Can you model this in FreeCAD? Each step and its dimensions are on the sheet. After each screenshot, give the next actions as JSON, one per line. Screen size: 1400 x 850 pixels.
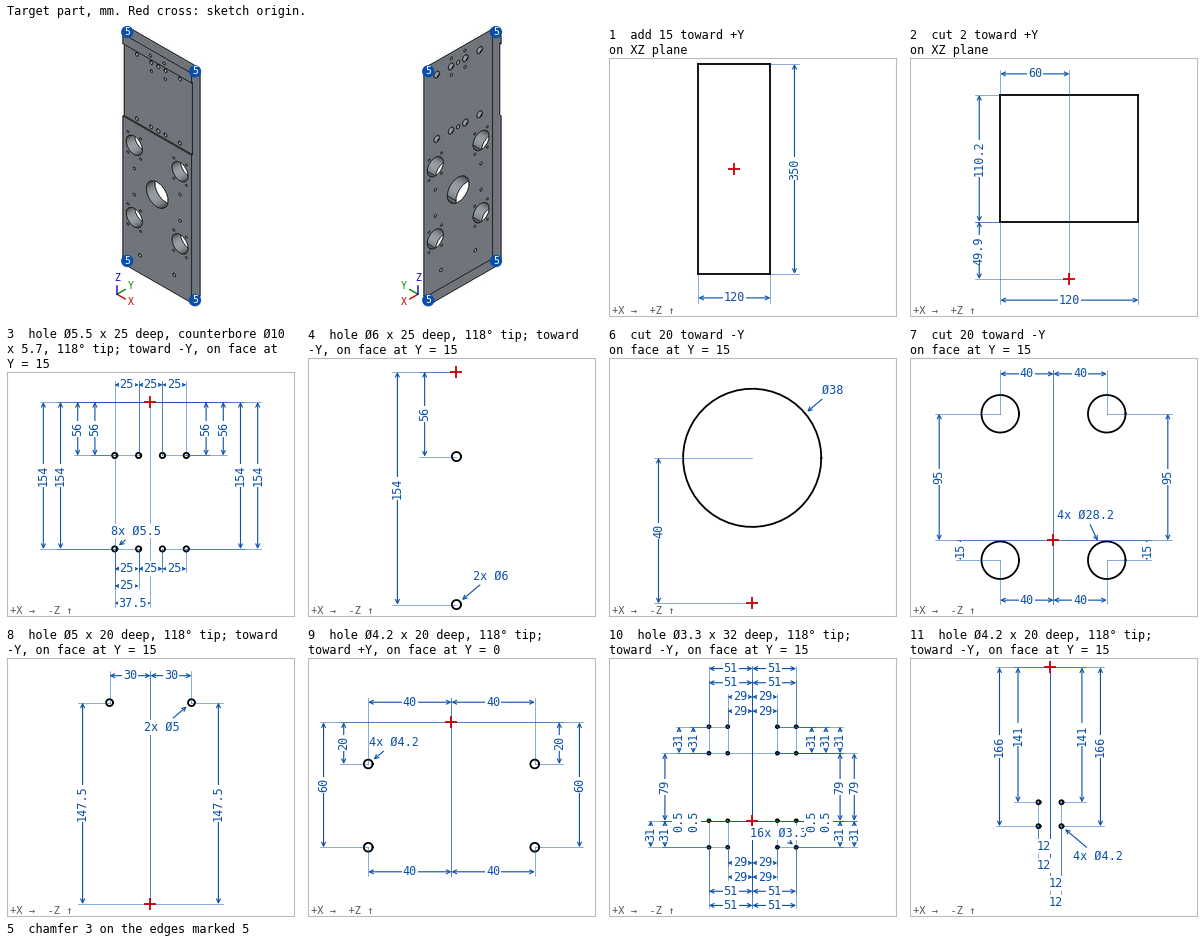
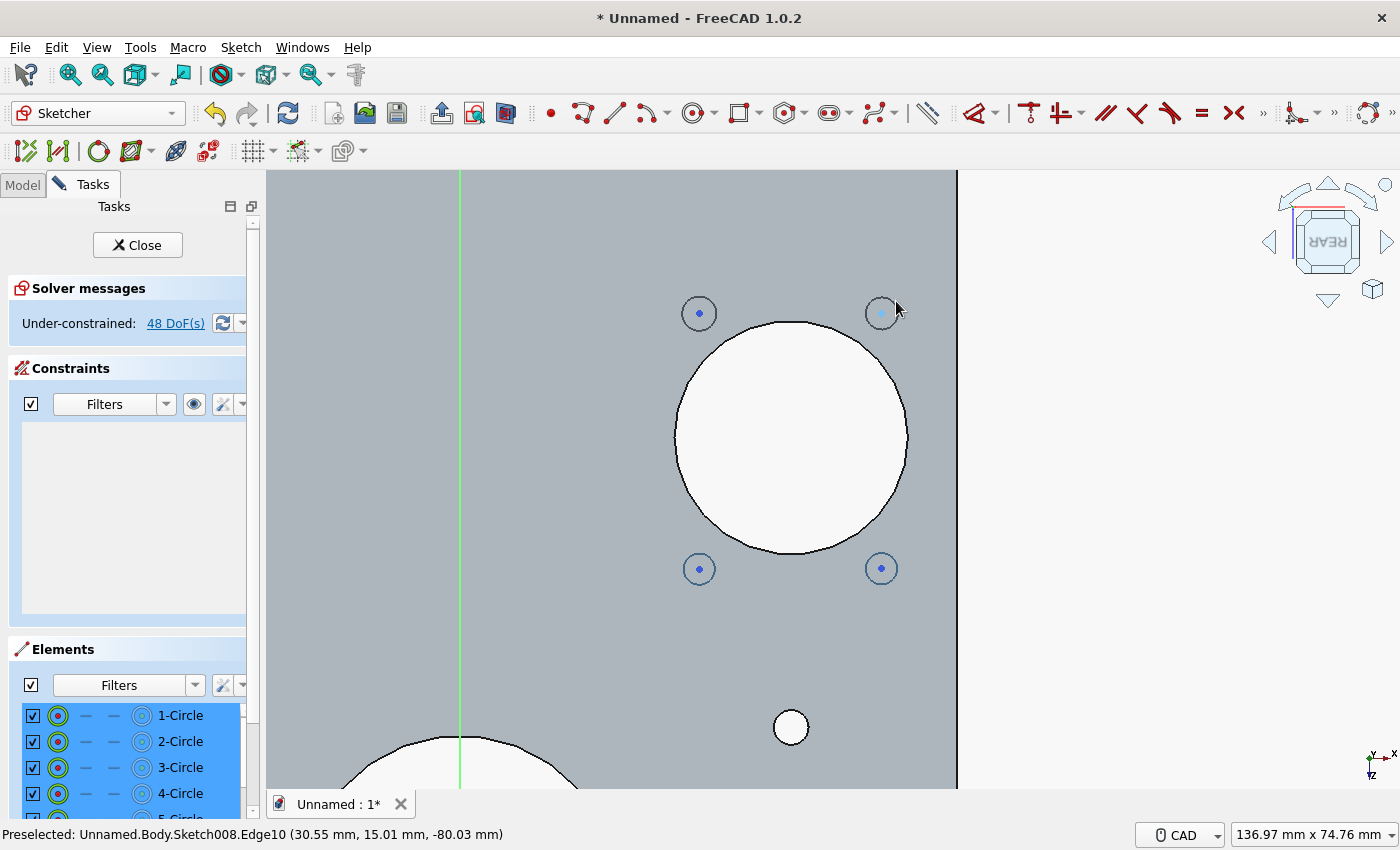
{"action": "left_click", "coordinate": [893, 302]}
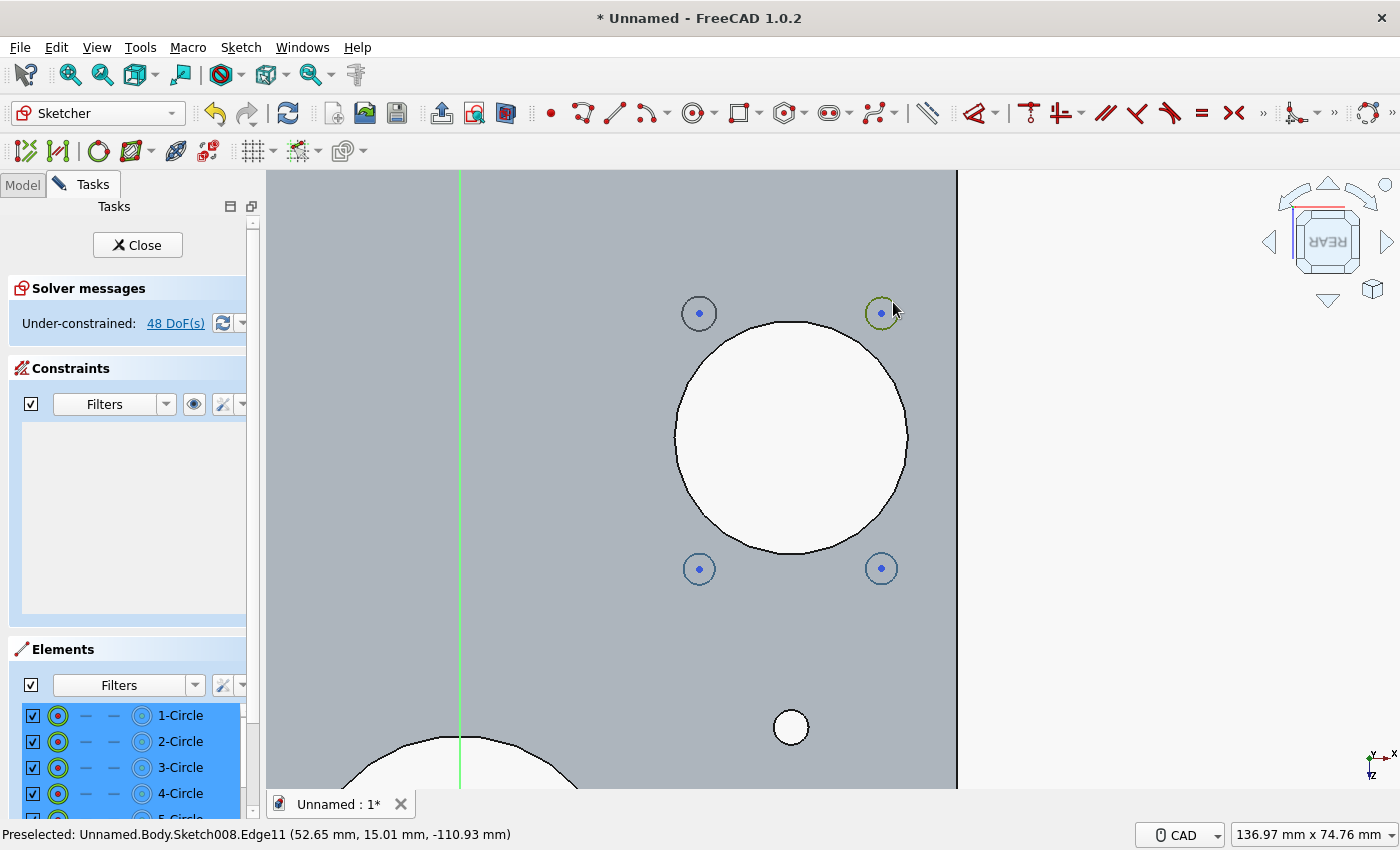
{"action": "left_click", "coordinate": [711, 302]}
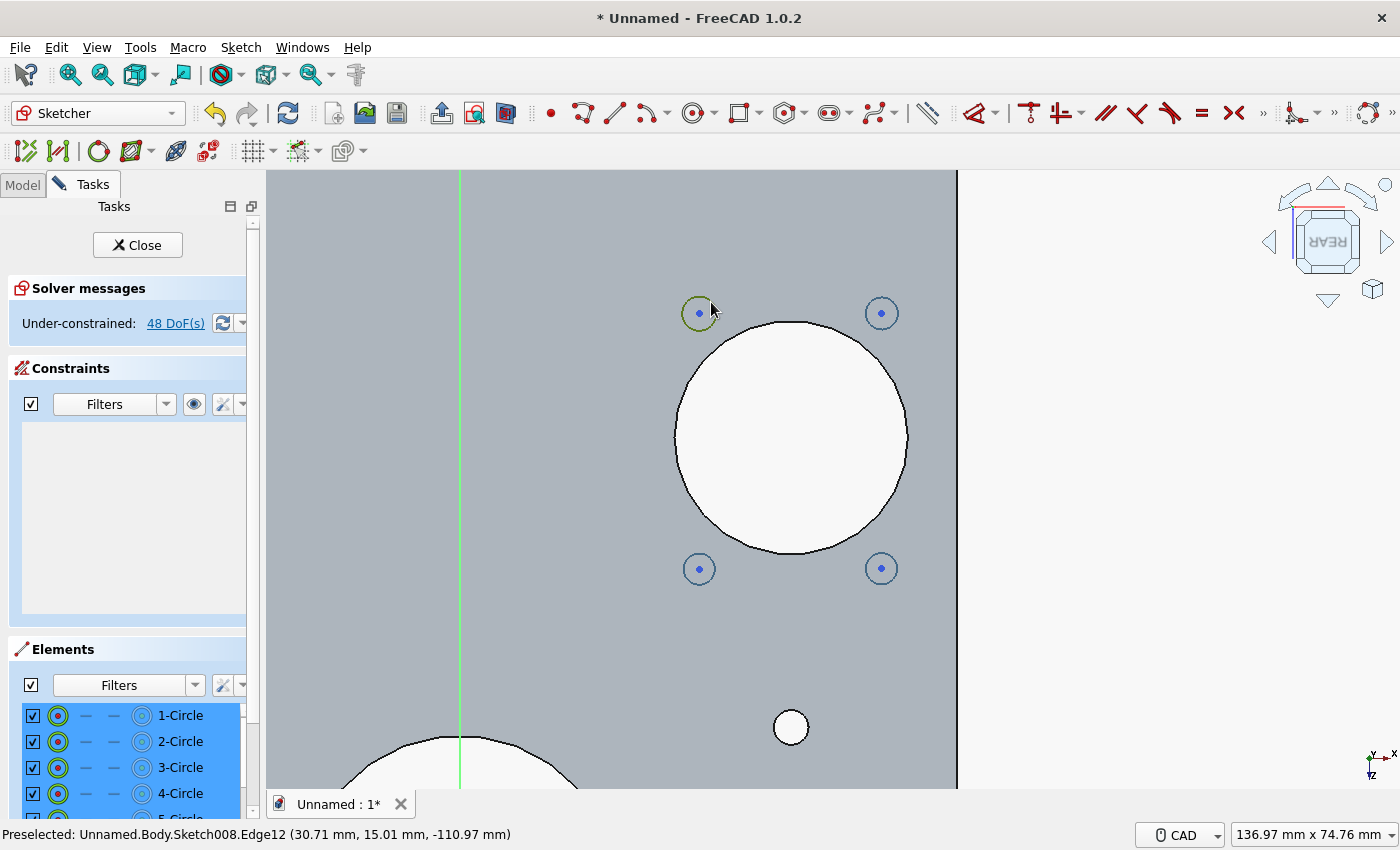
{"action": "scroll", "coordinate": [896, 301], "scroll_direction": "down", "scroll_amount": 6}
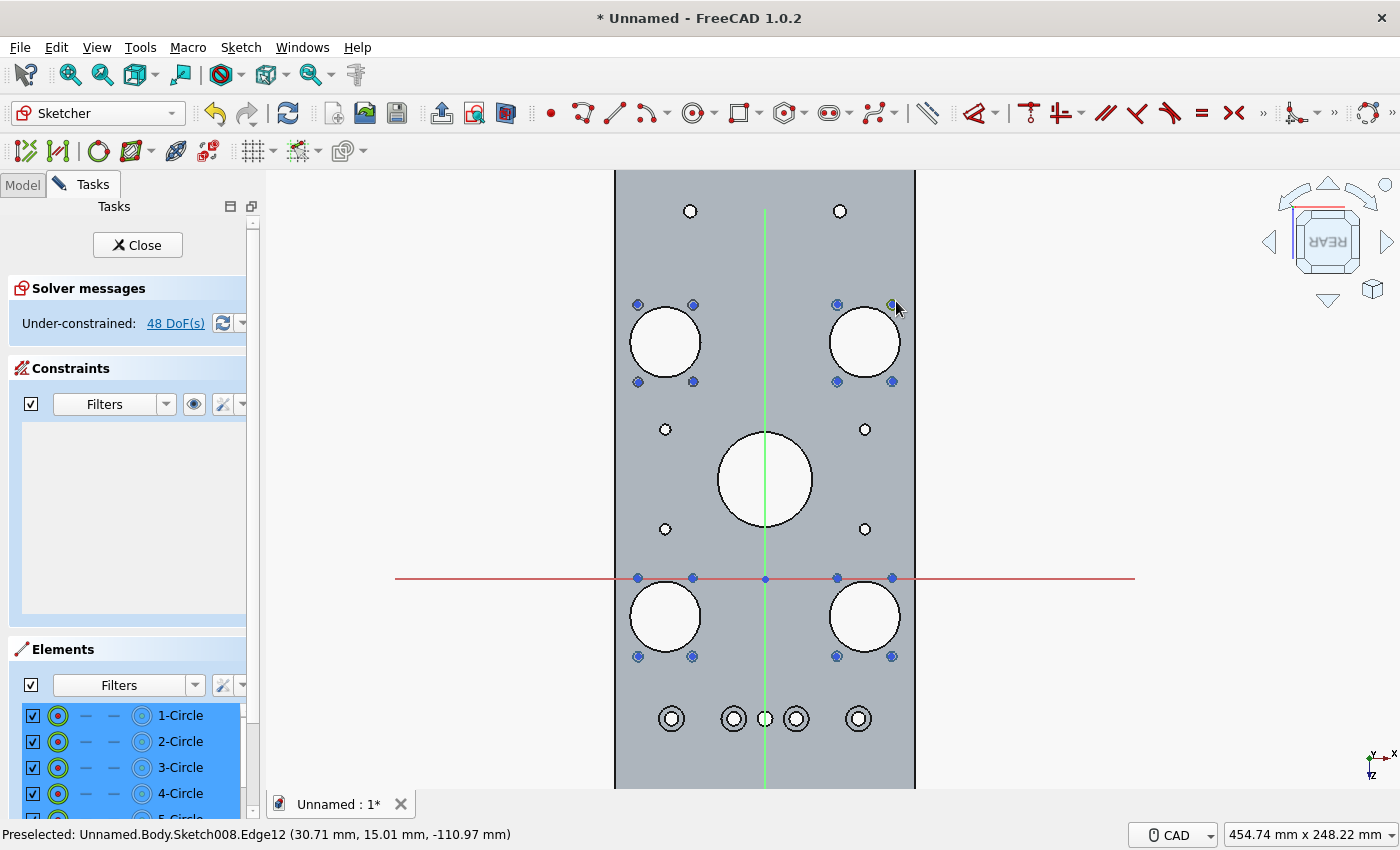
{"action": "scroll", "coordinate": [696, 379], "scroll_direction": "up", "scroll_amount": 6}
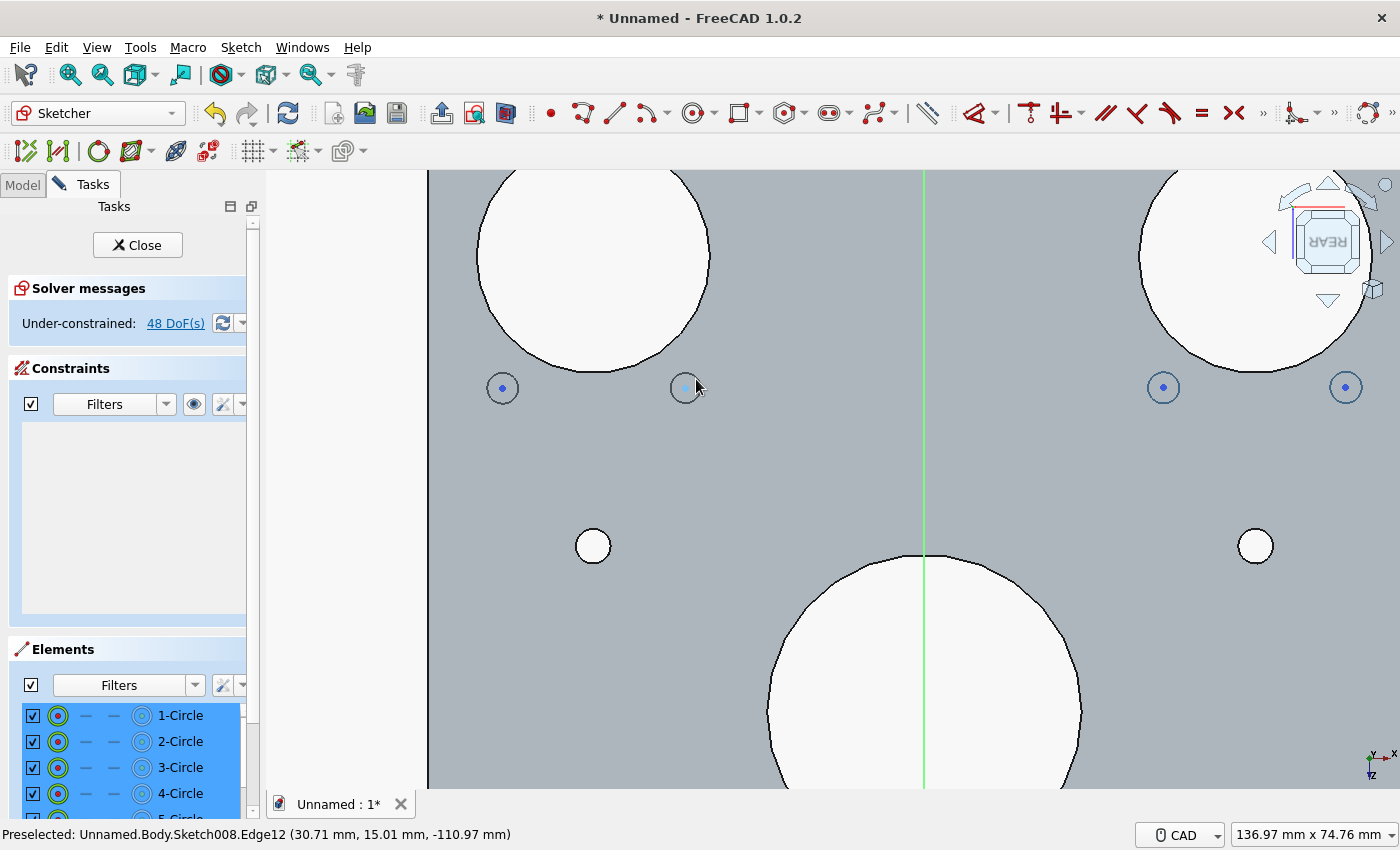
{"action": "left_click", "coordinate": [696, 377]}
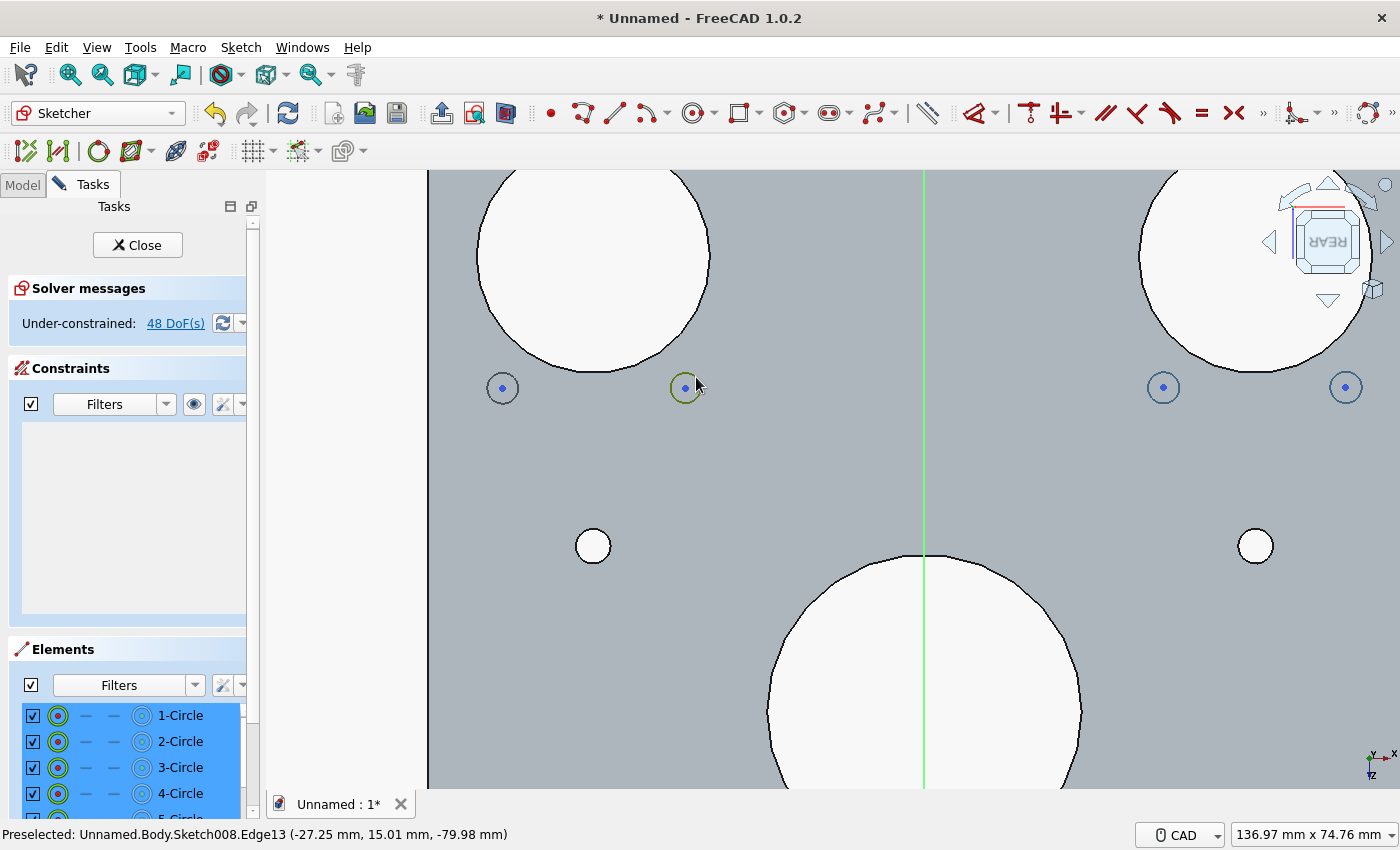
{"action": "left_click", "coordinate": [514, 377]}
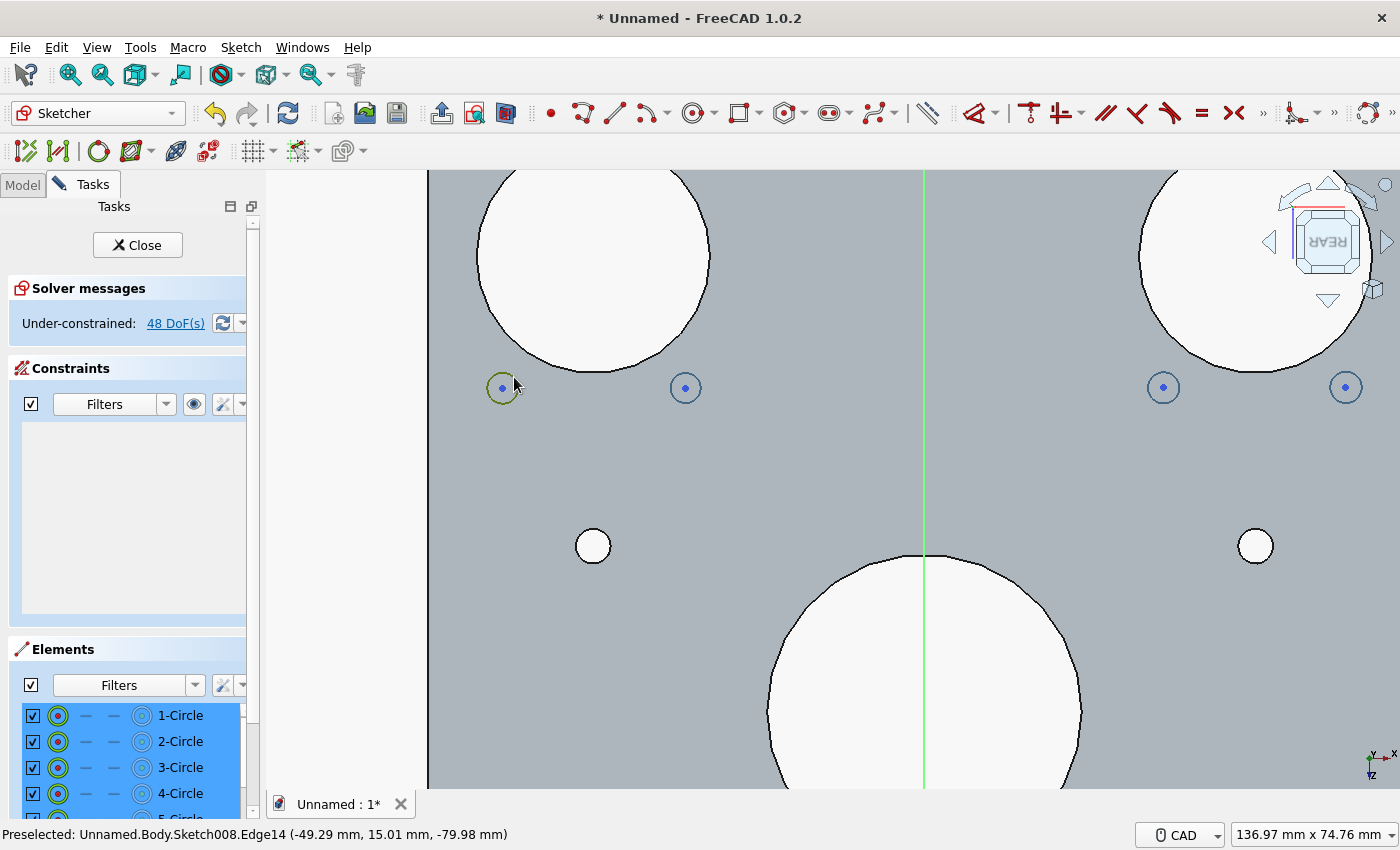
{"action": "scroll", "coordinate": [696, 379], "scroll_direction": "down", "scroll_amount": 6}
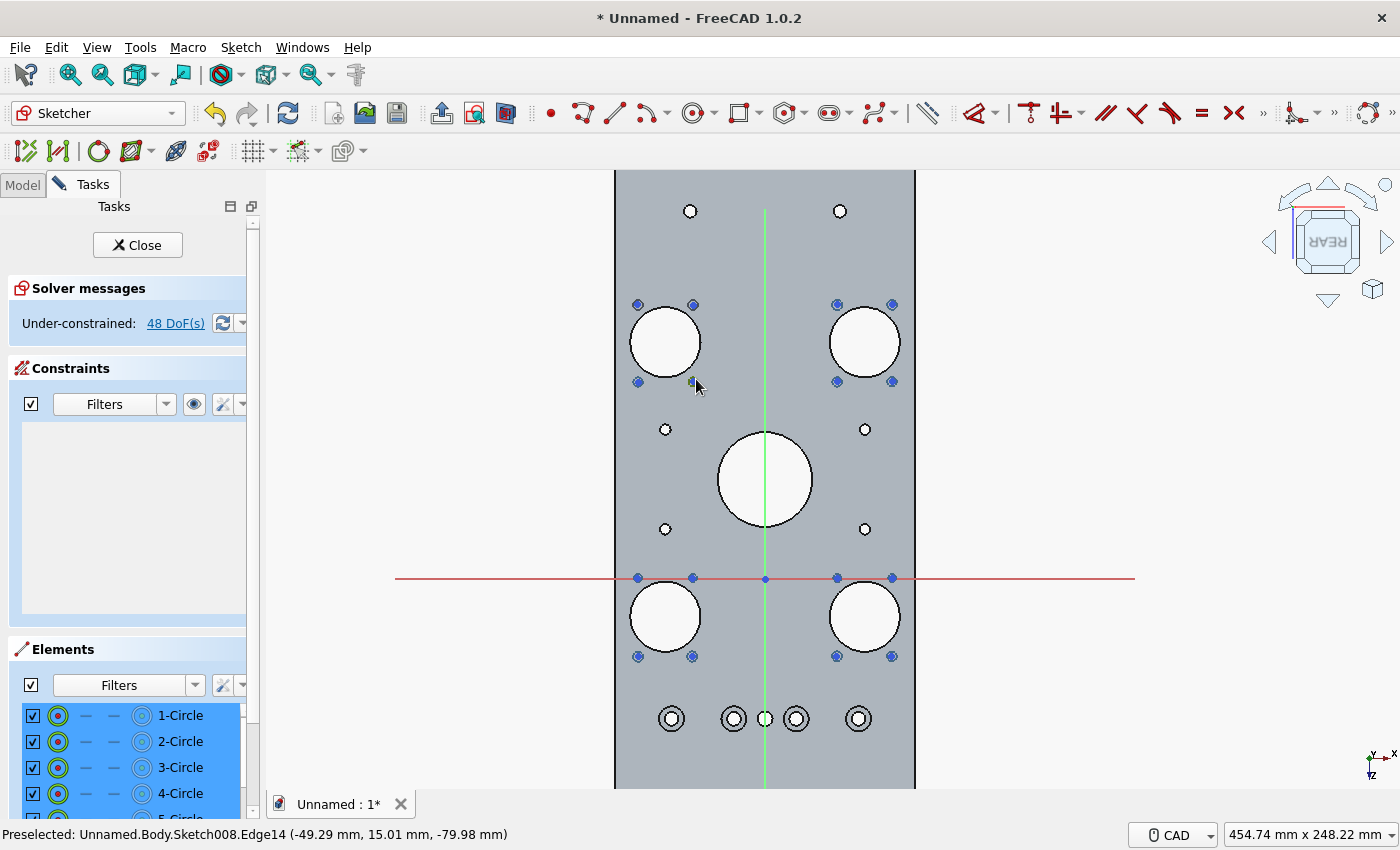
{"action": "scroll", "coordinate": [696, 302], "scroll_direction": "up", "scroll_amount": 6}